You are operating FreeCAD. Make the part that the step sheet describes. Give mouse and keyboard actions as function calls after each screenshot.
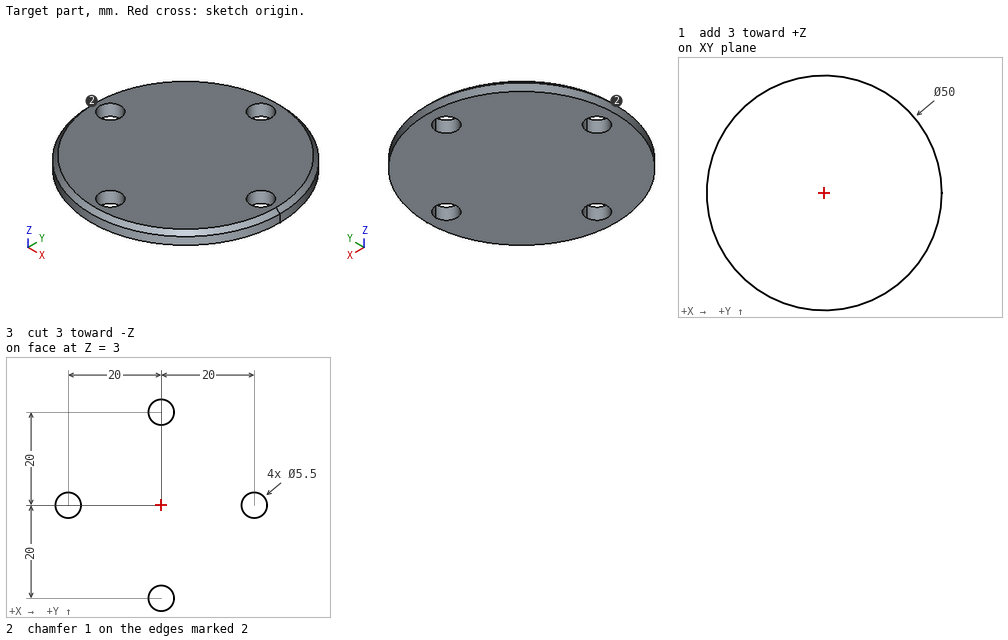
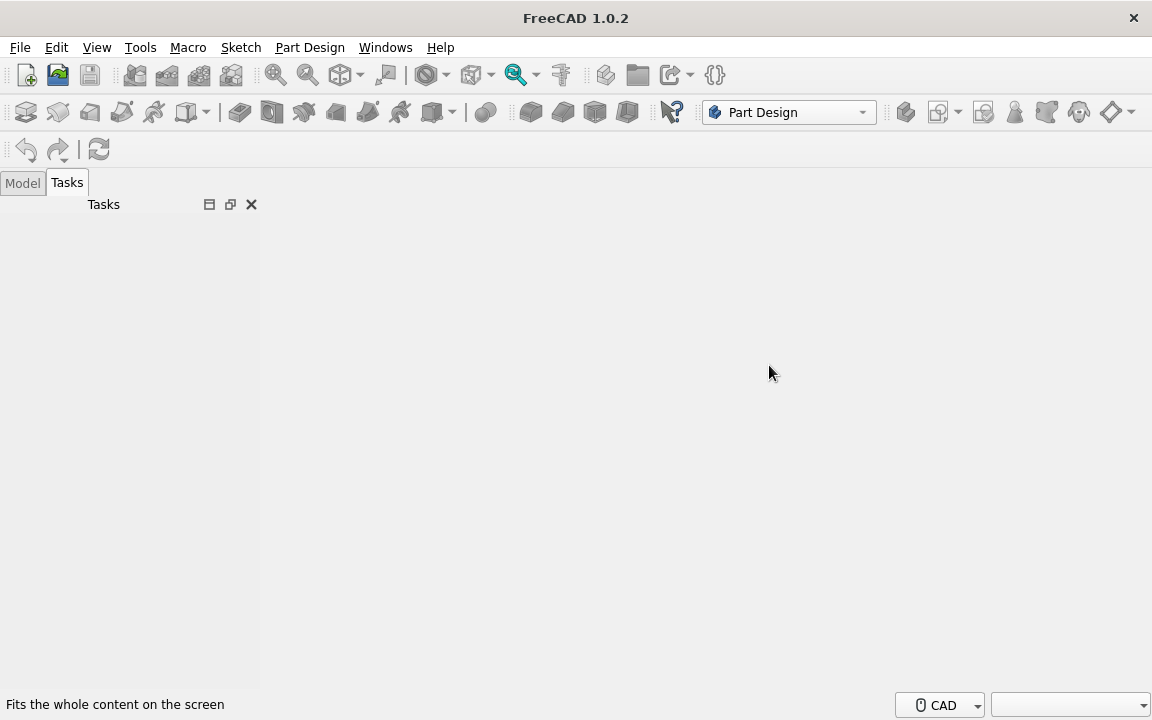
click(26, 76)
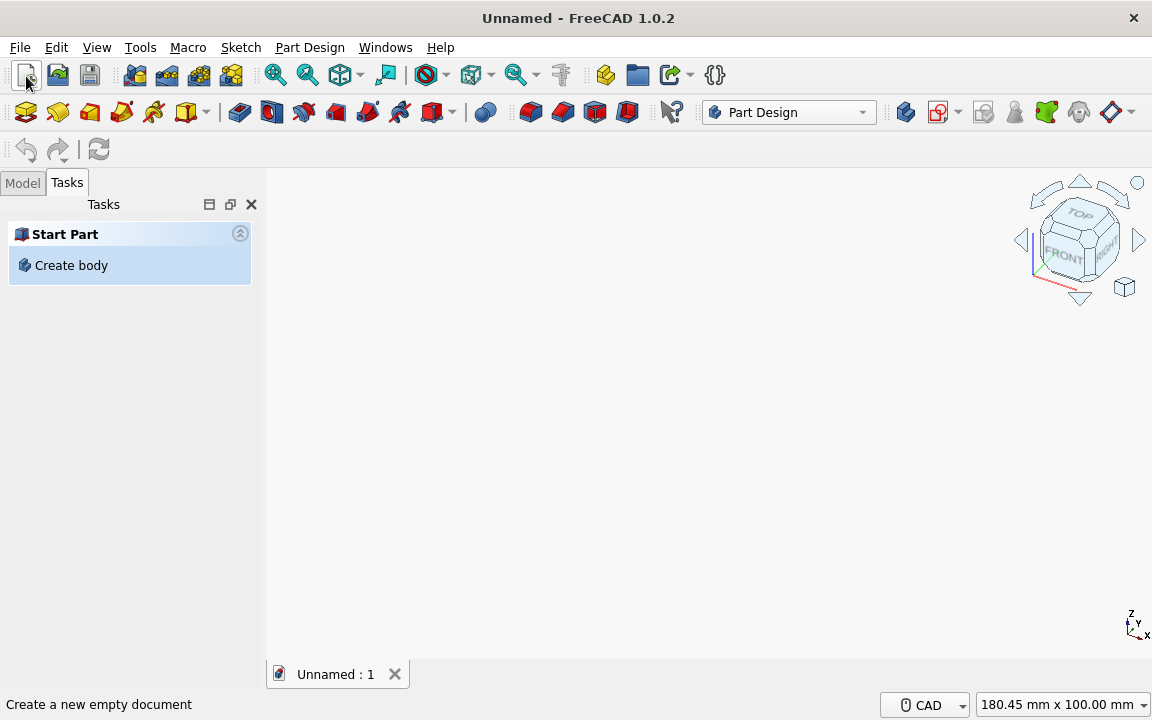
click(938, 112)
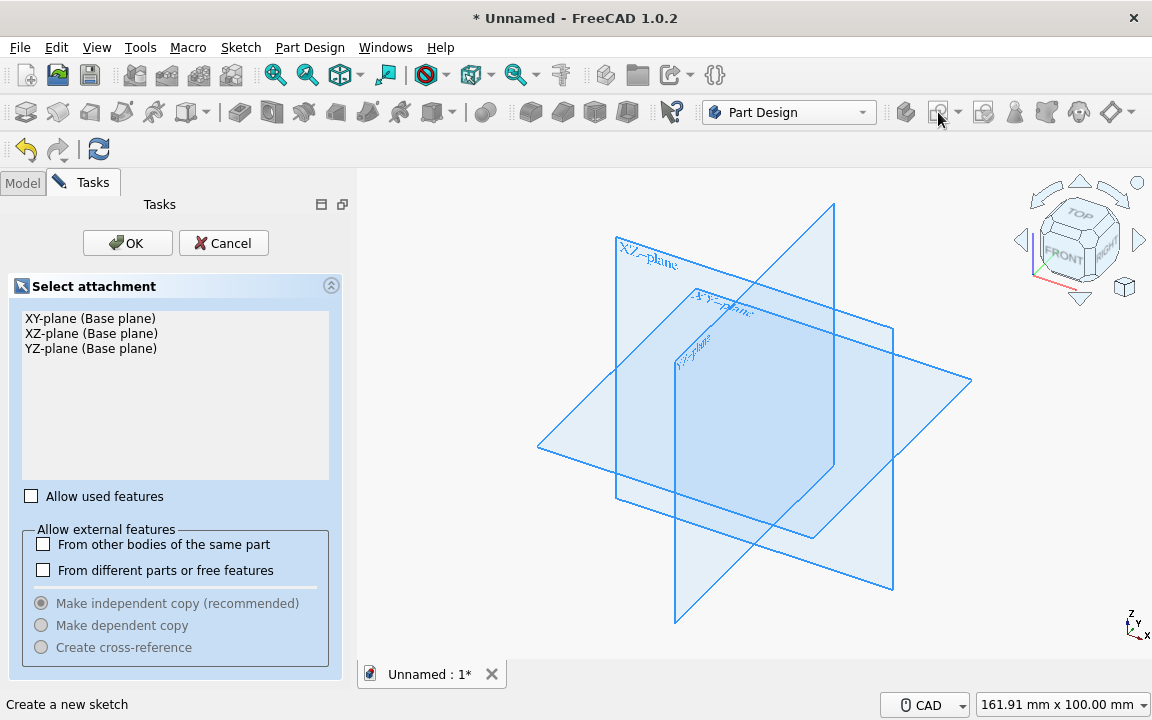
click(82, 318)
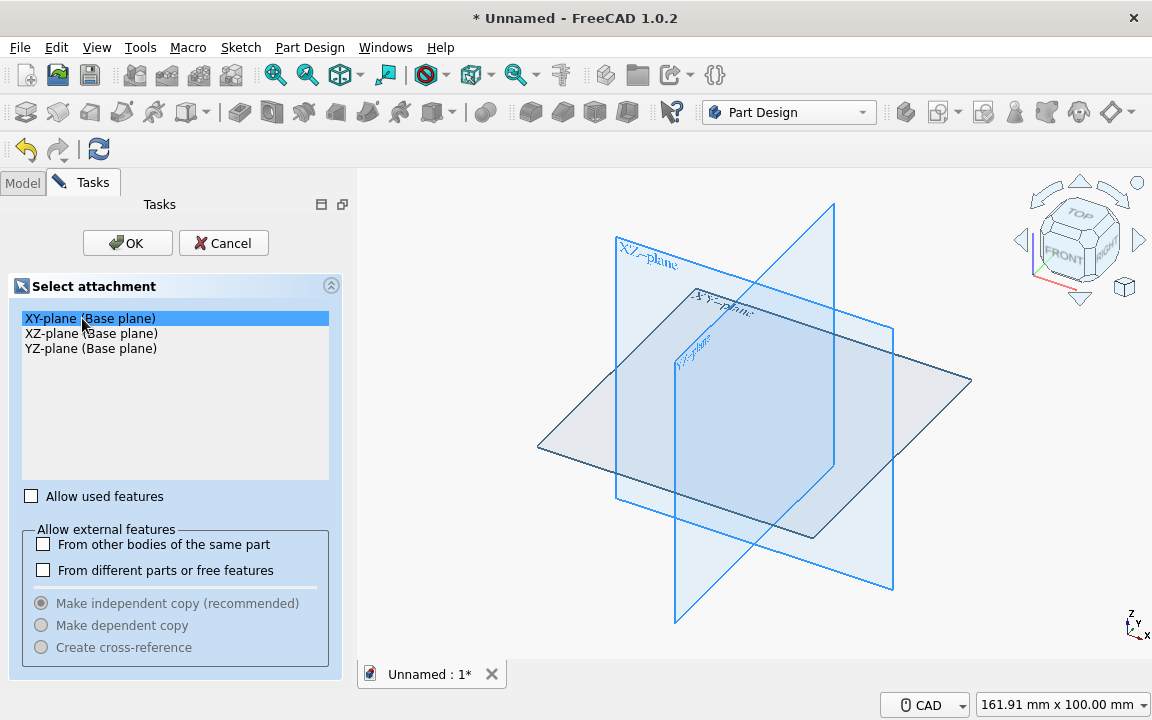
click(128, 243)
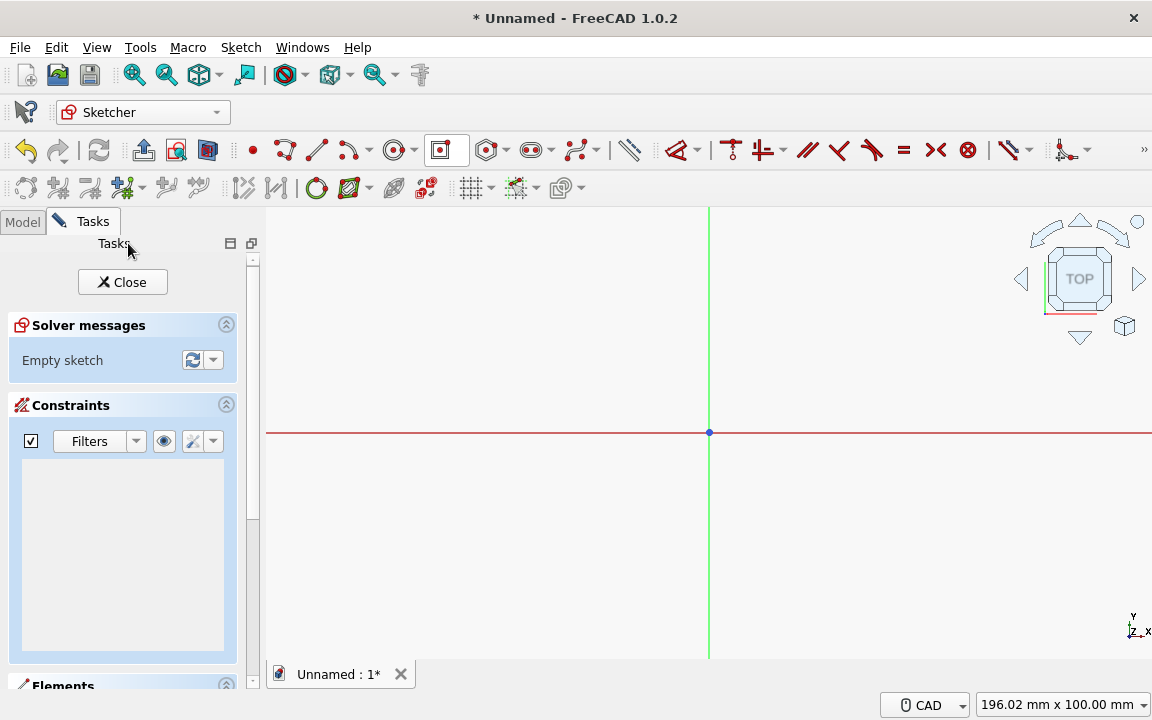
click(394, 150)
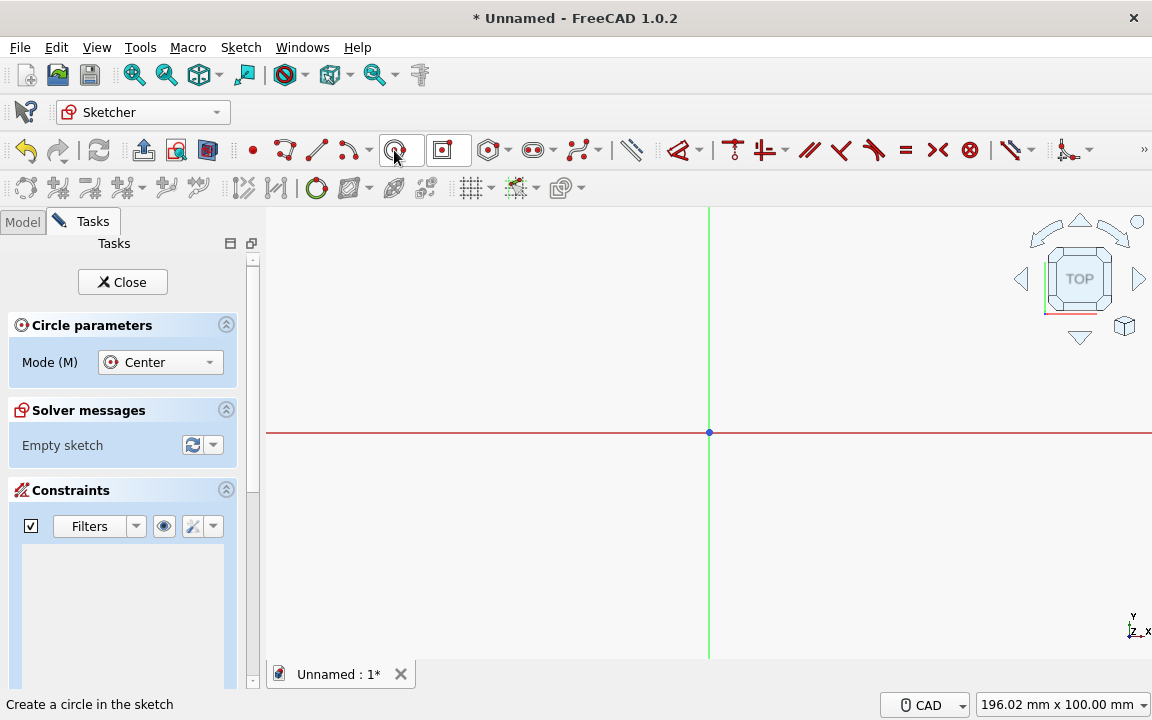
click(709, 433)
move(789, 353)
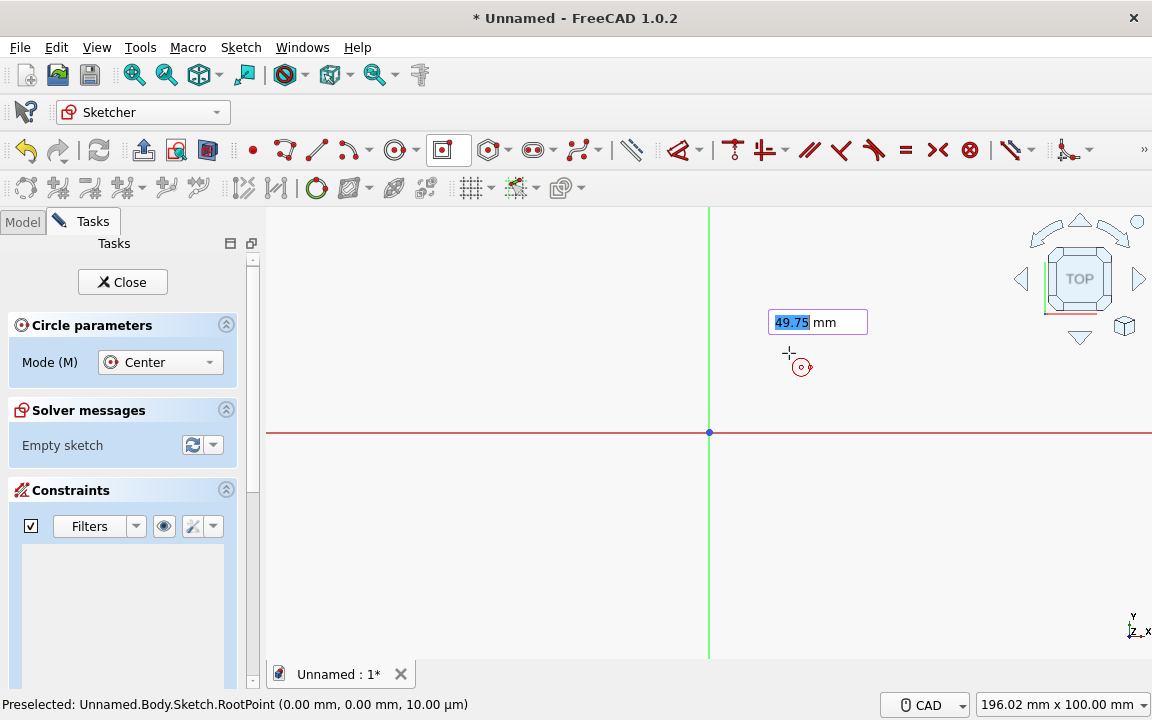
text(50)
key(Return)
key(Escape)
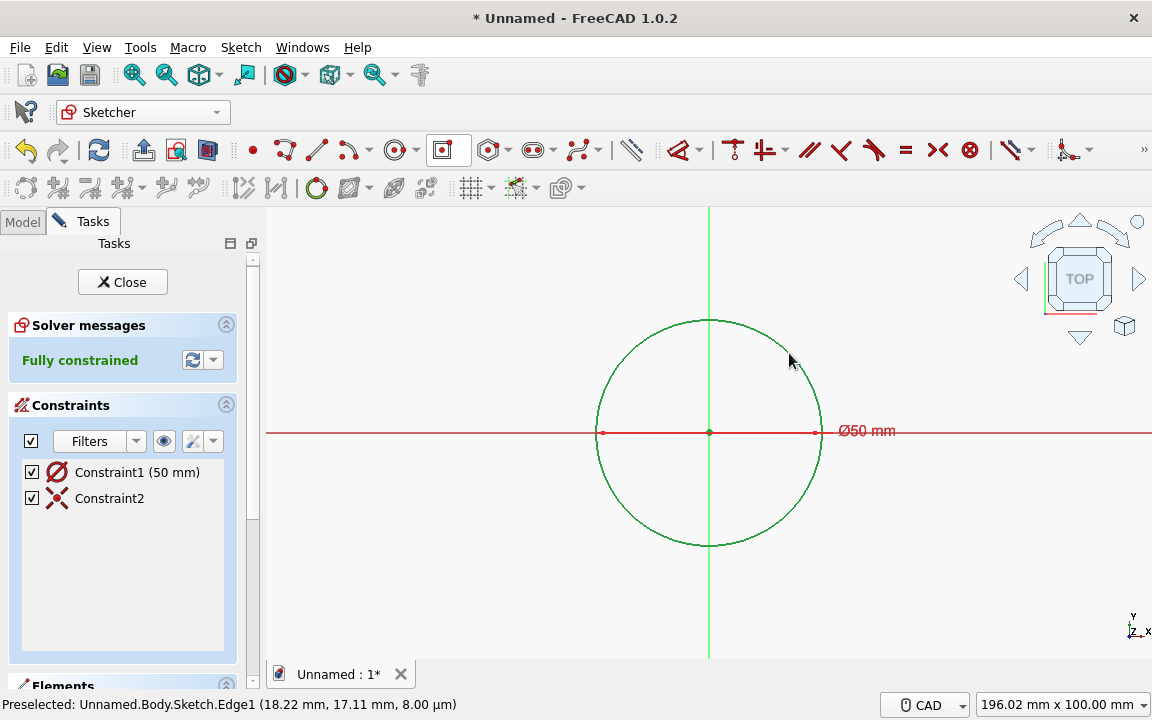
click(123, 282)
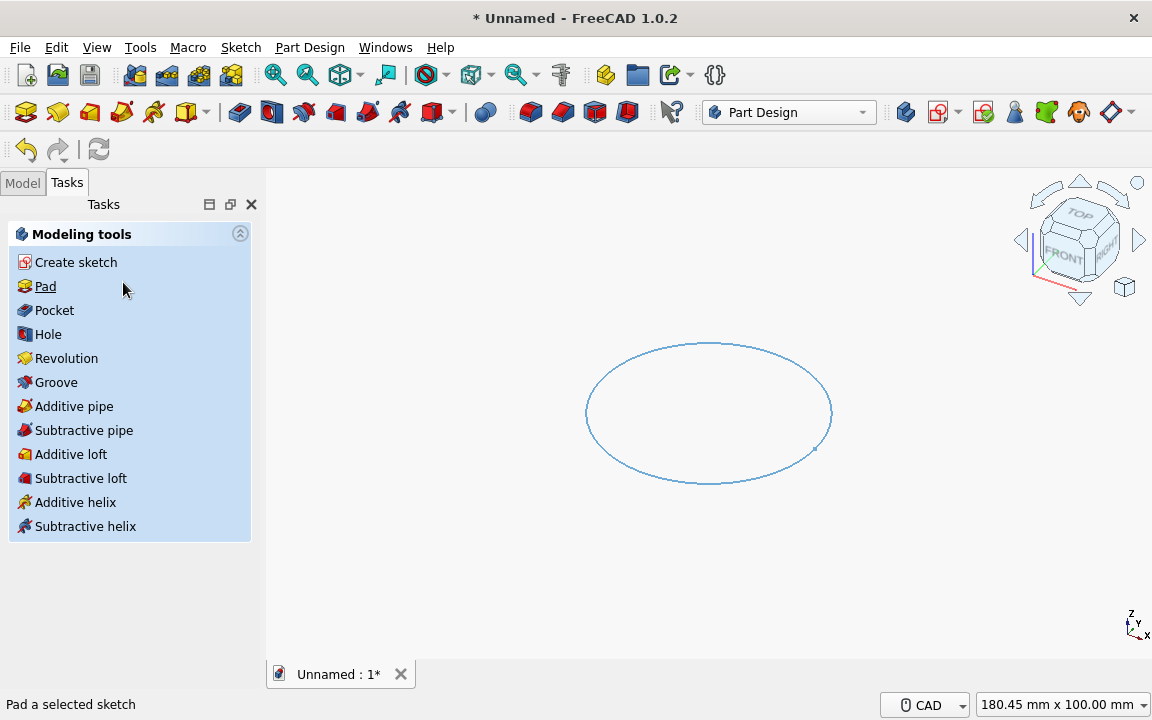
click(26, 112)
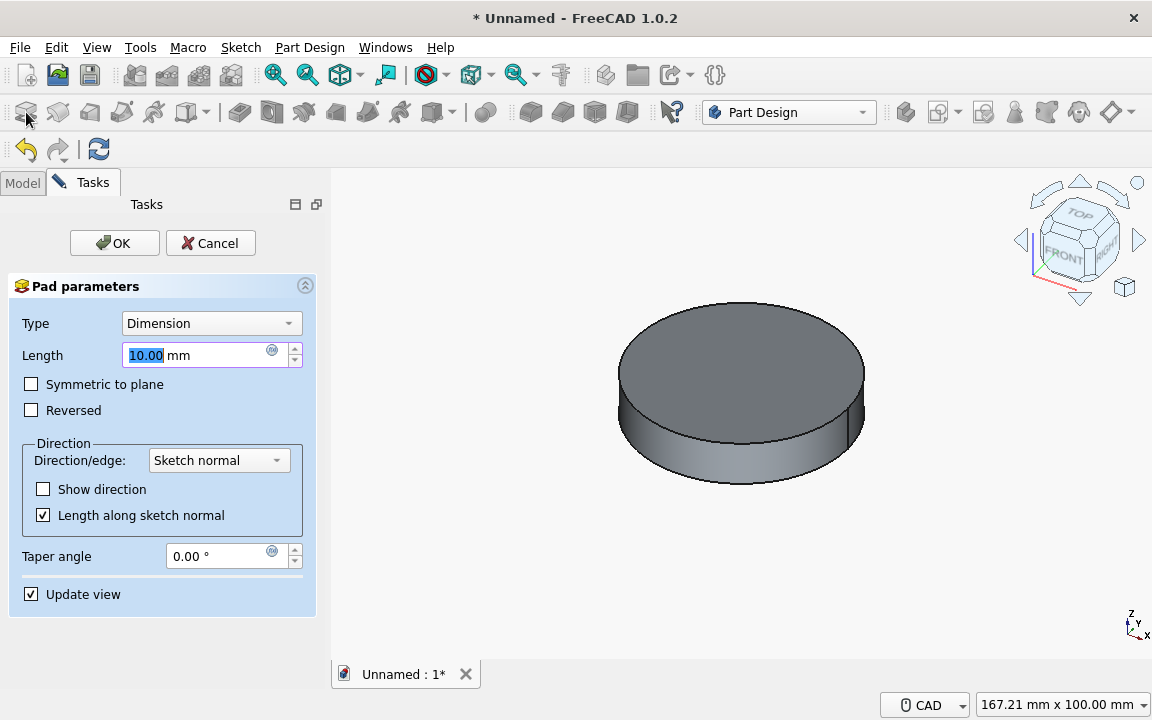
text(3)
key(Tab)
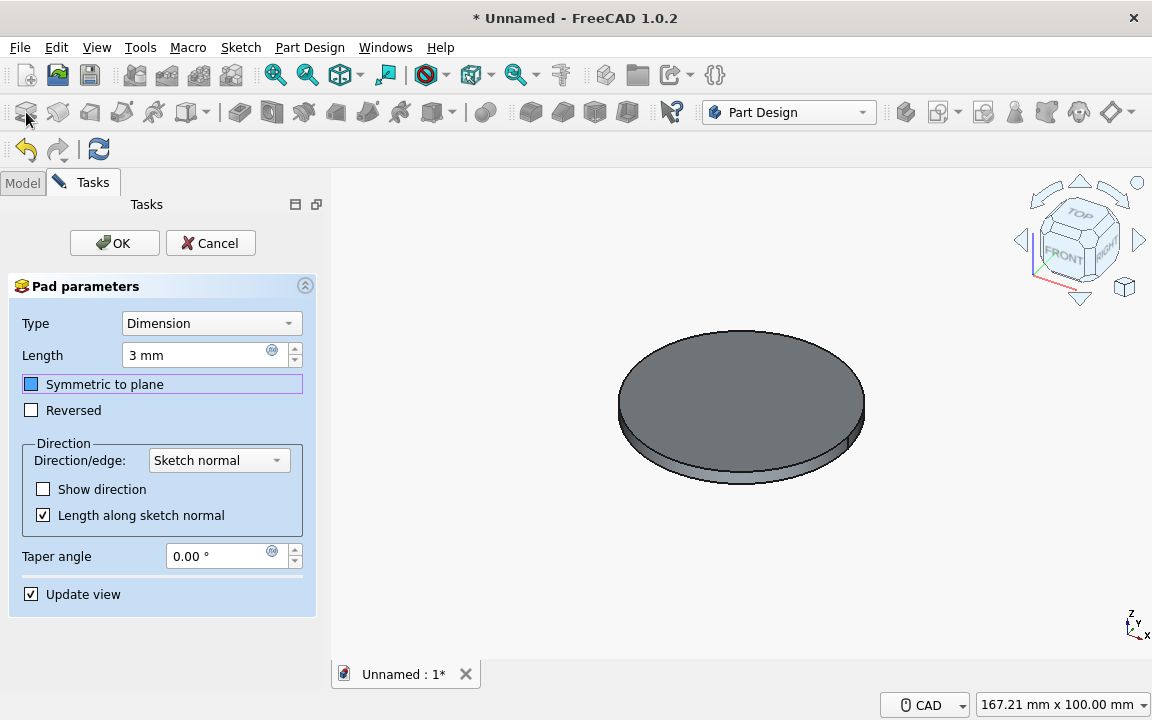
click(115, 243)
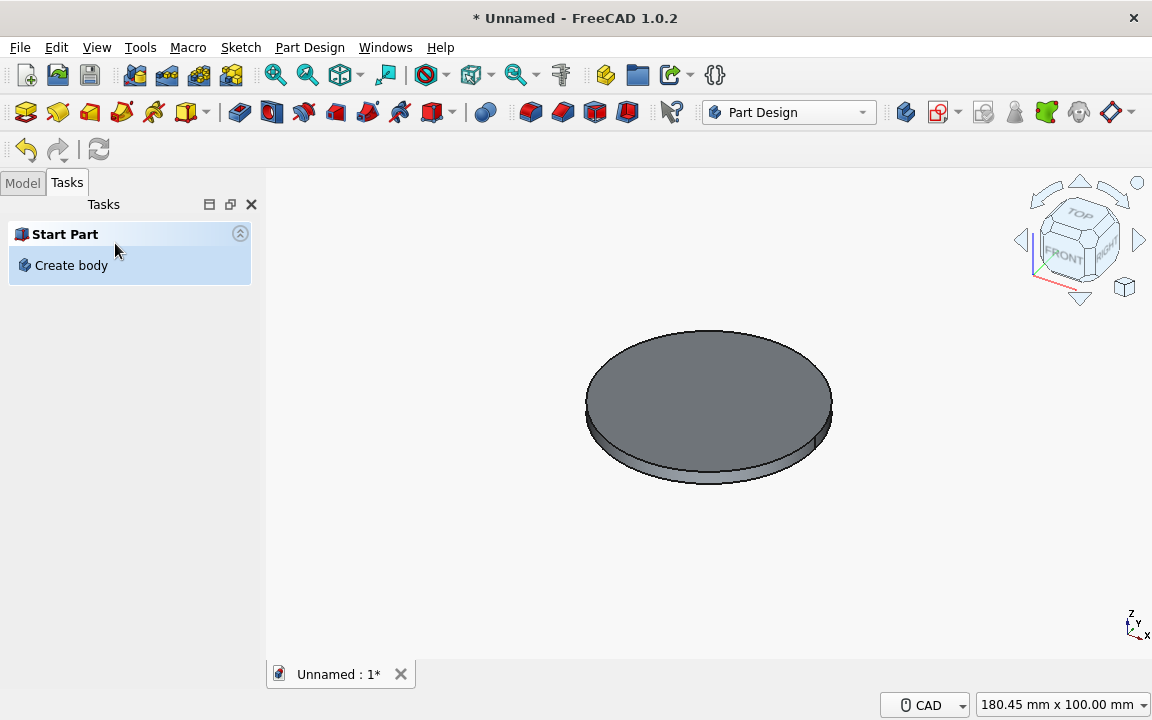
key(v)
key(f)